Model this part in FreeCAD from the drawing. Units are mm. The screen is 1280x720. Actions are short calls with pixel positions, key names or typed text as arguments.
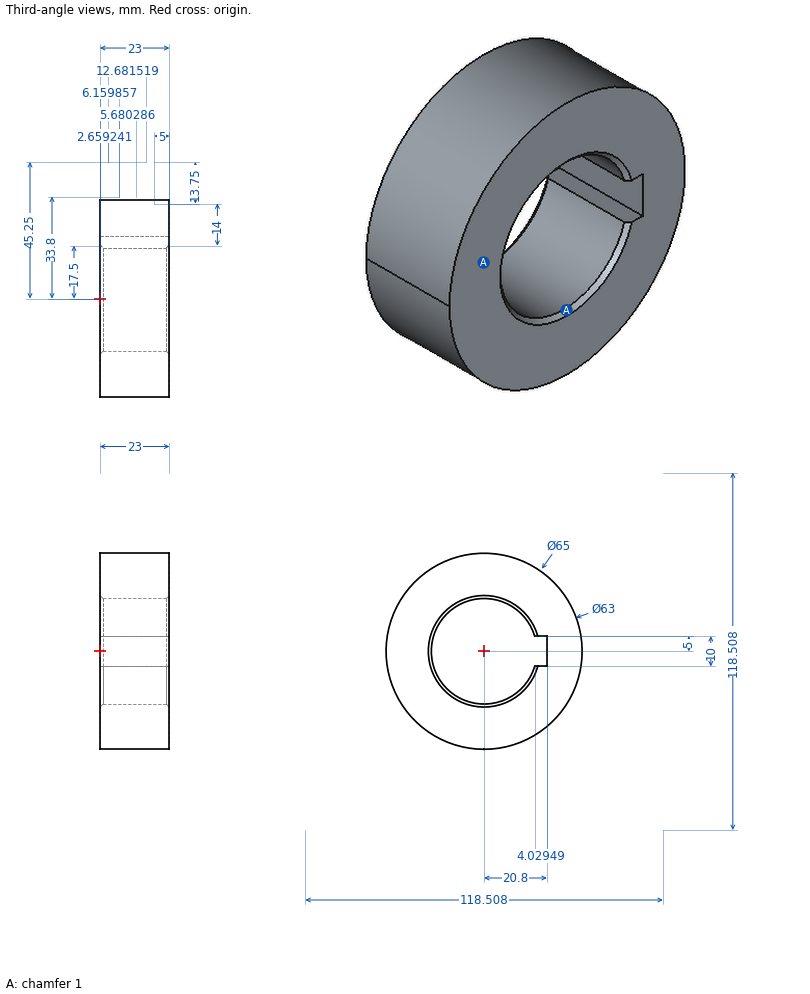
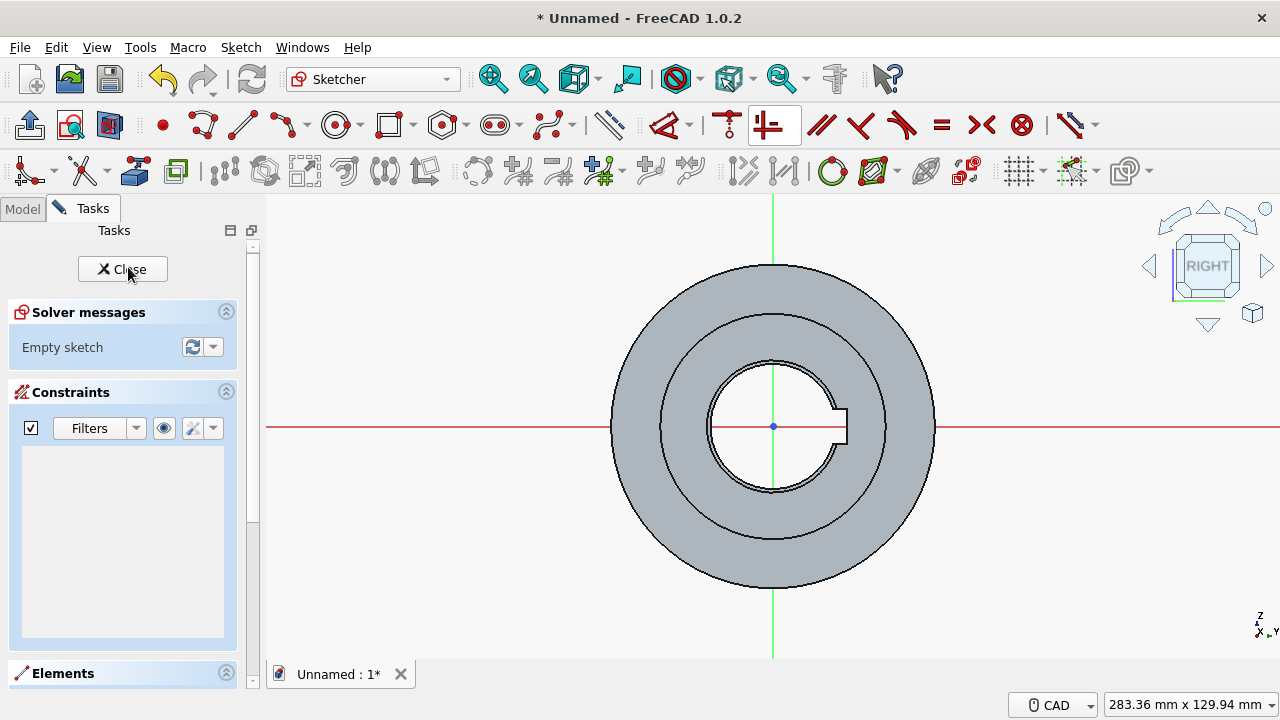
key(q)
key(s)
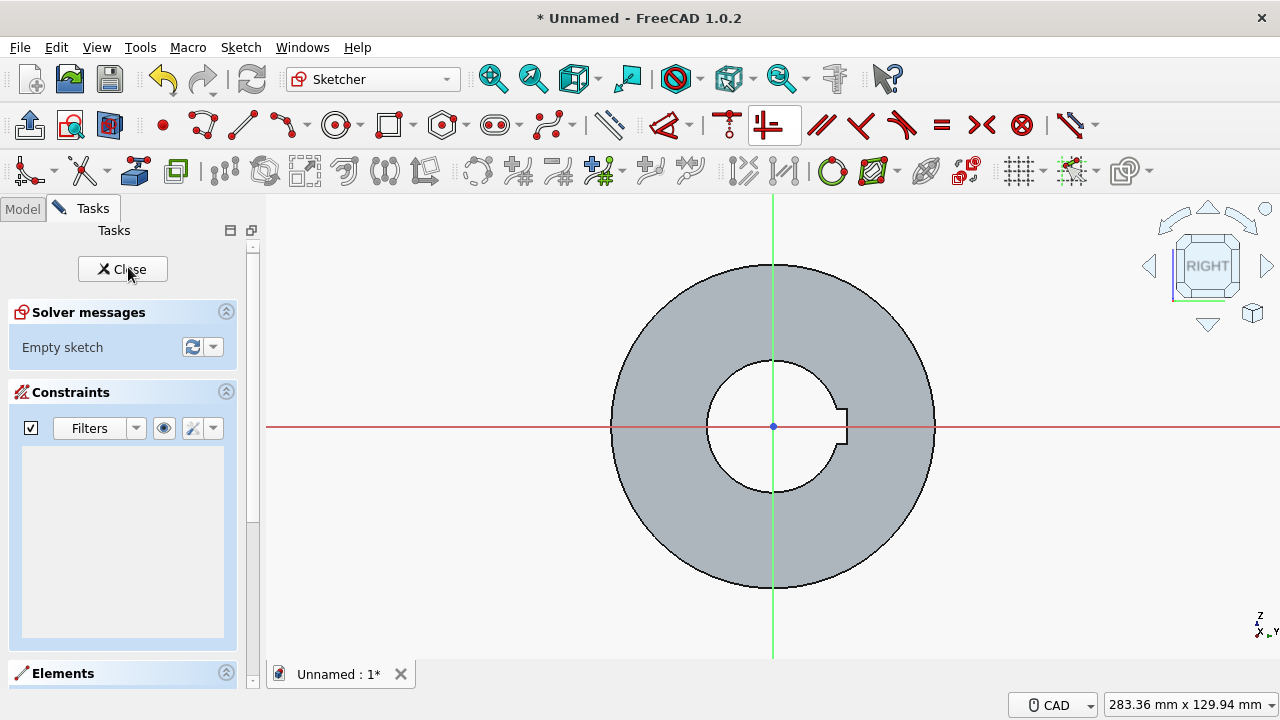
scroll(565, 426, down, 2)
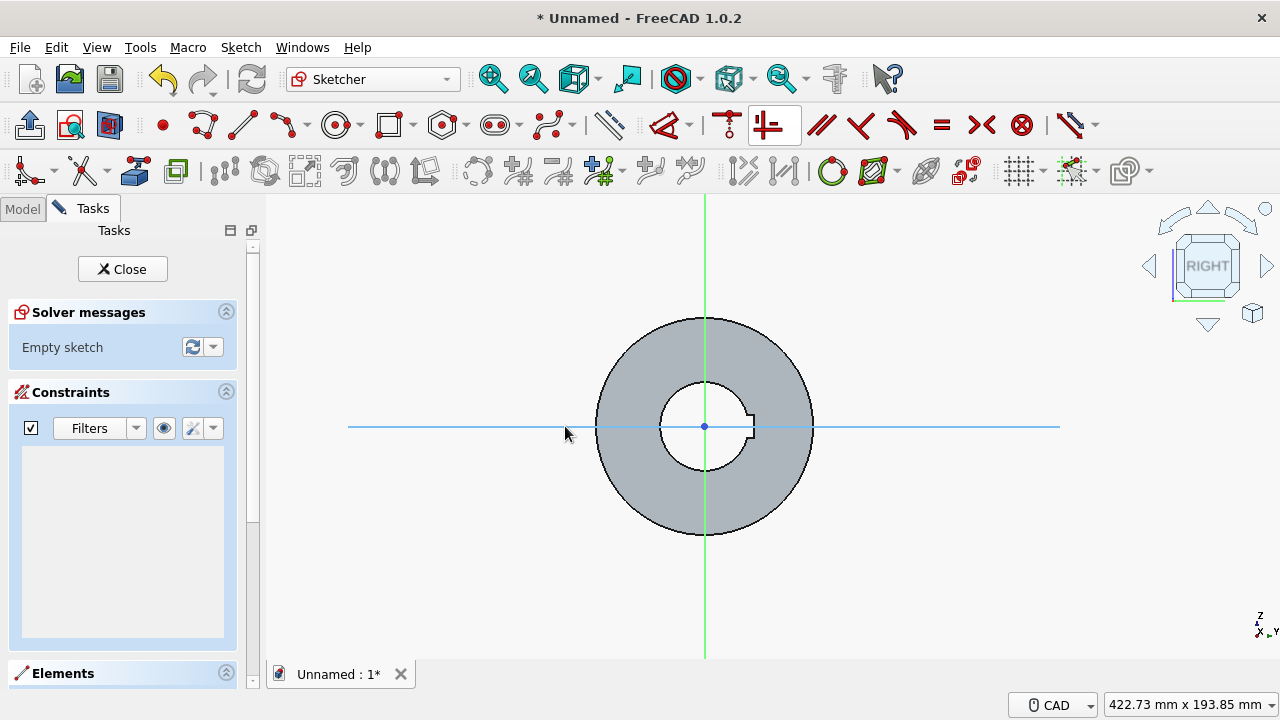
key(g)
key(v)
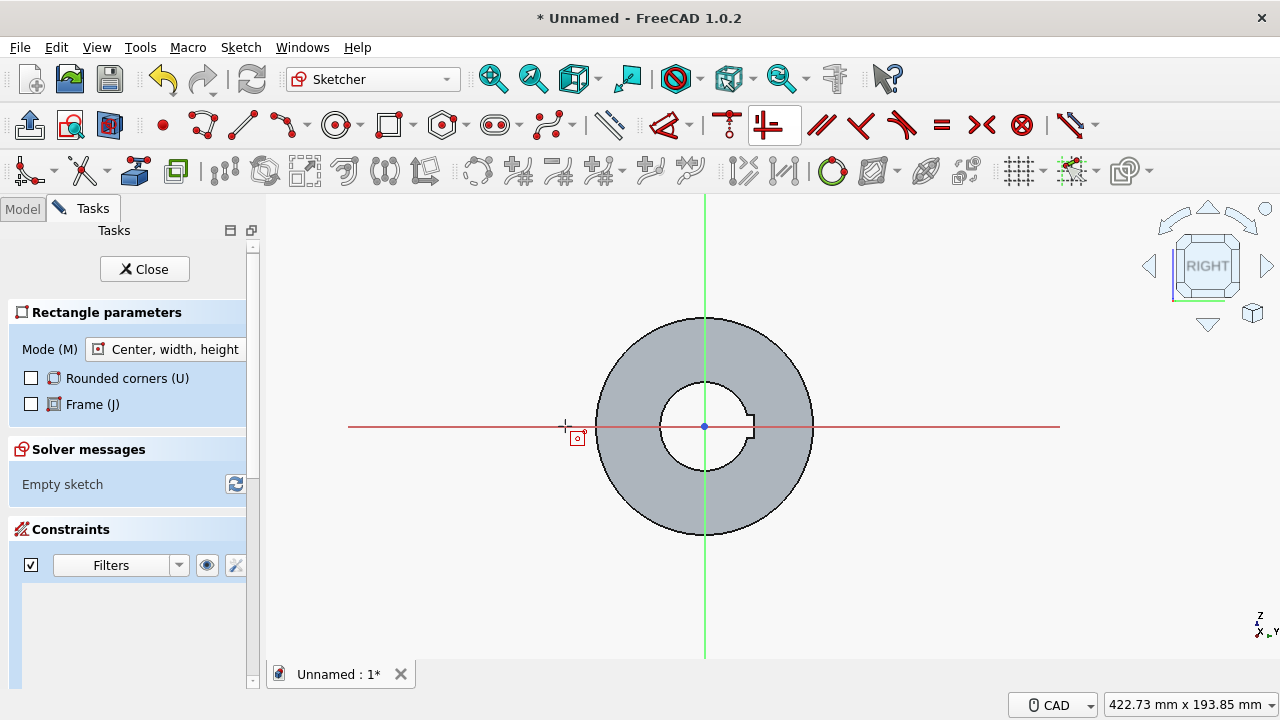
click(705, 427)
move(847, 284)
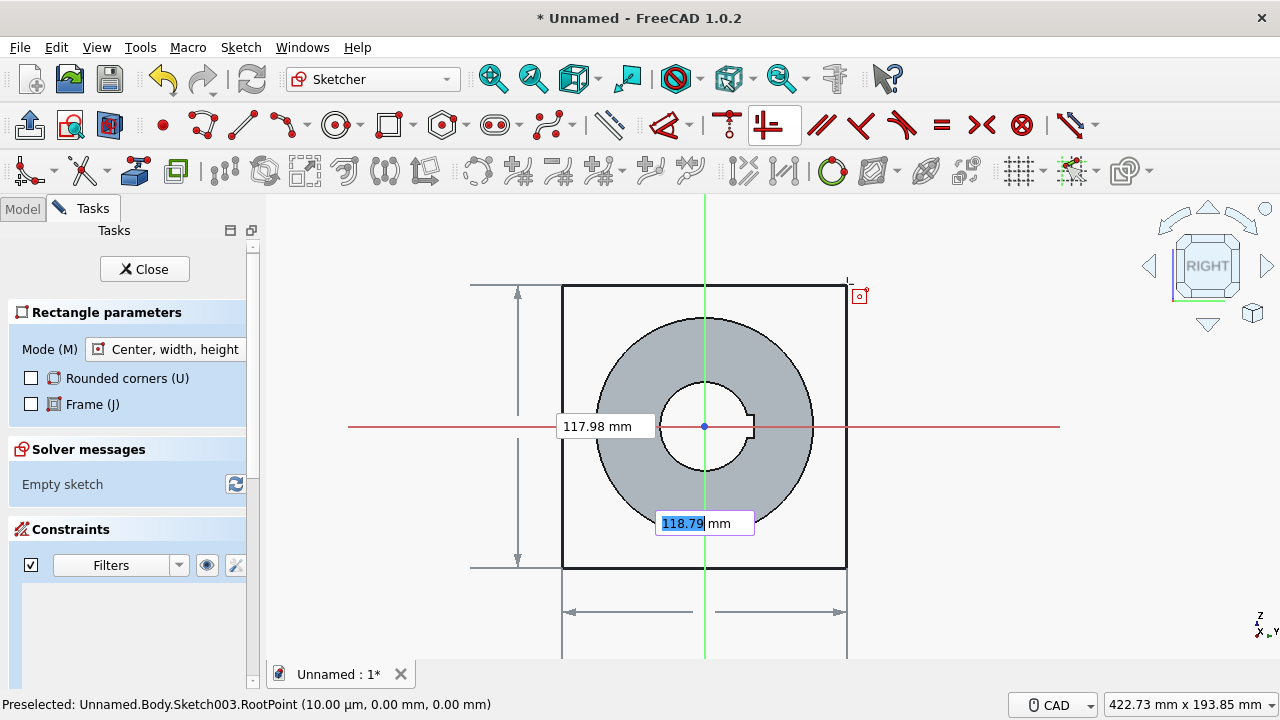
text(118.508)
key(Tab)
text(118.508)
key(Return)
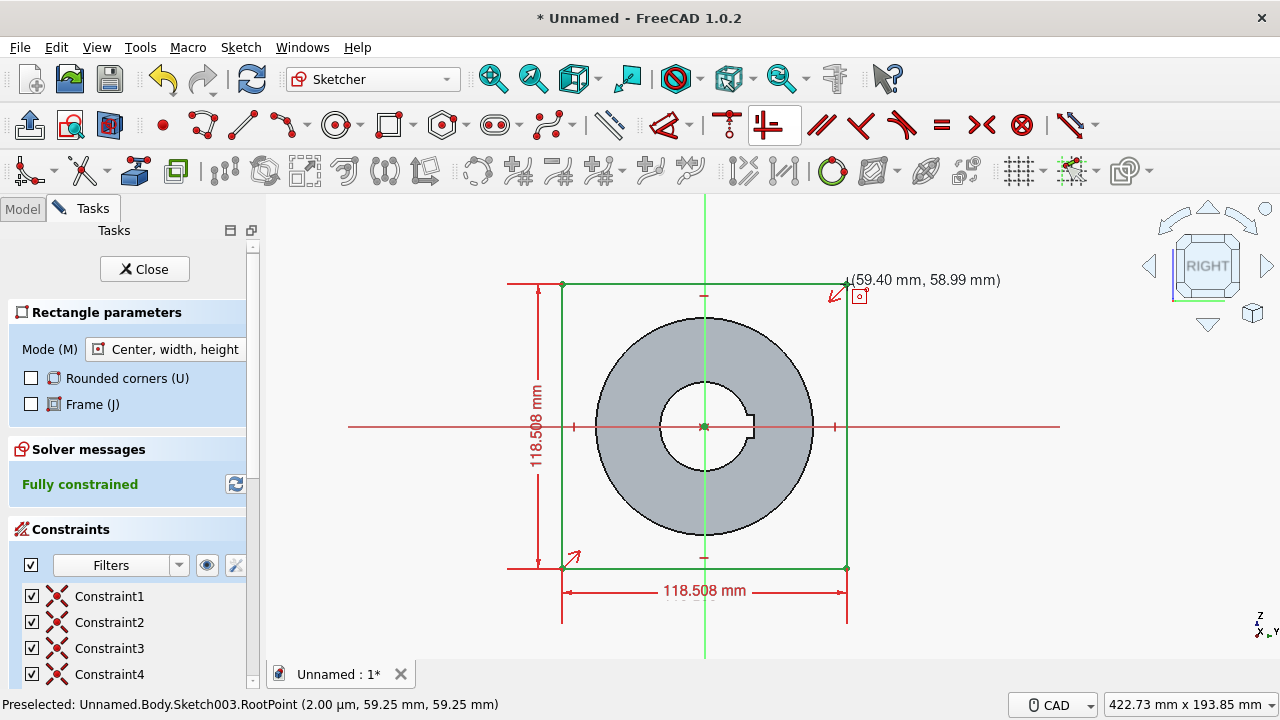
key(g)
key(c)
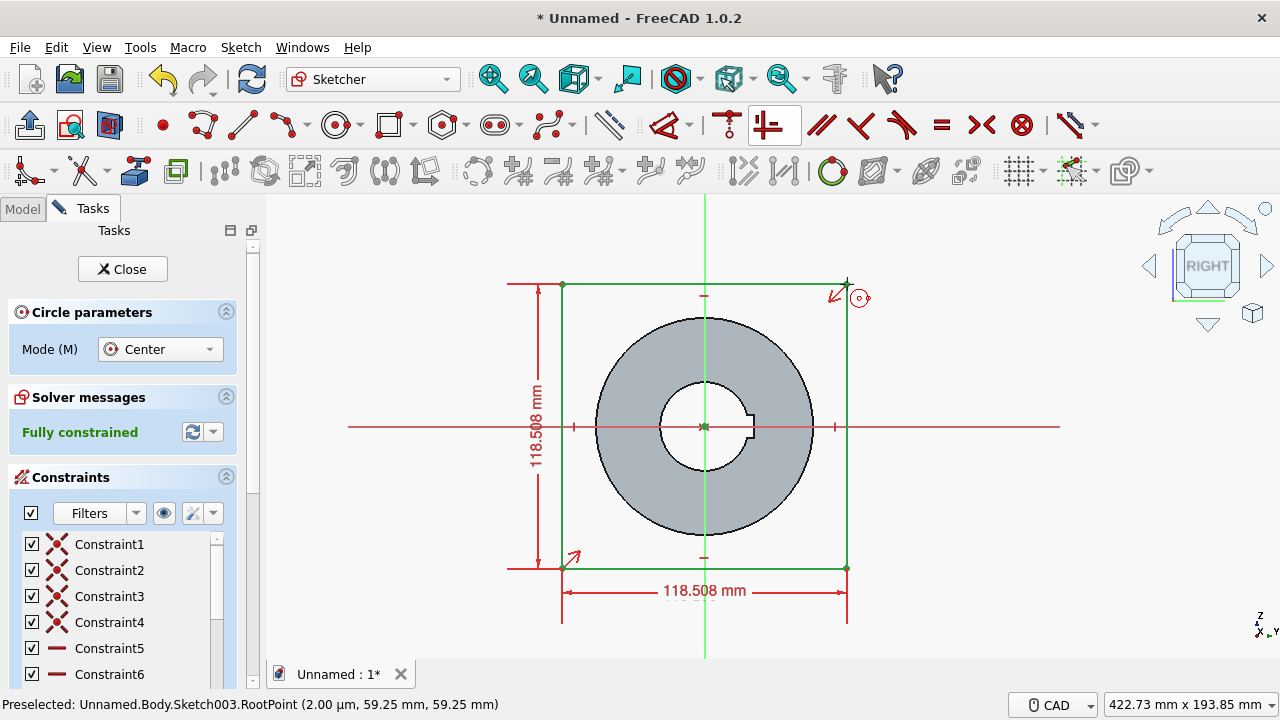
click(705, 427)
move(758, 373)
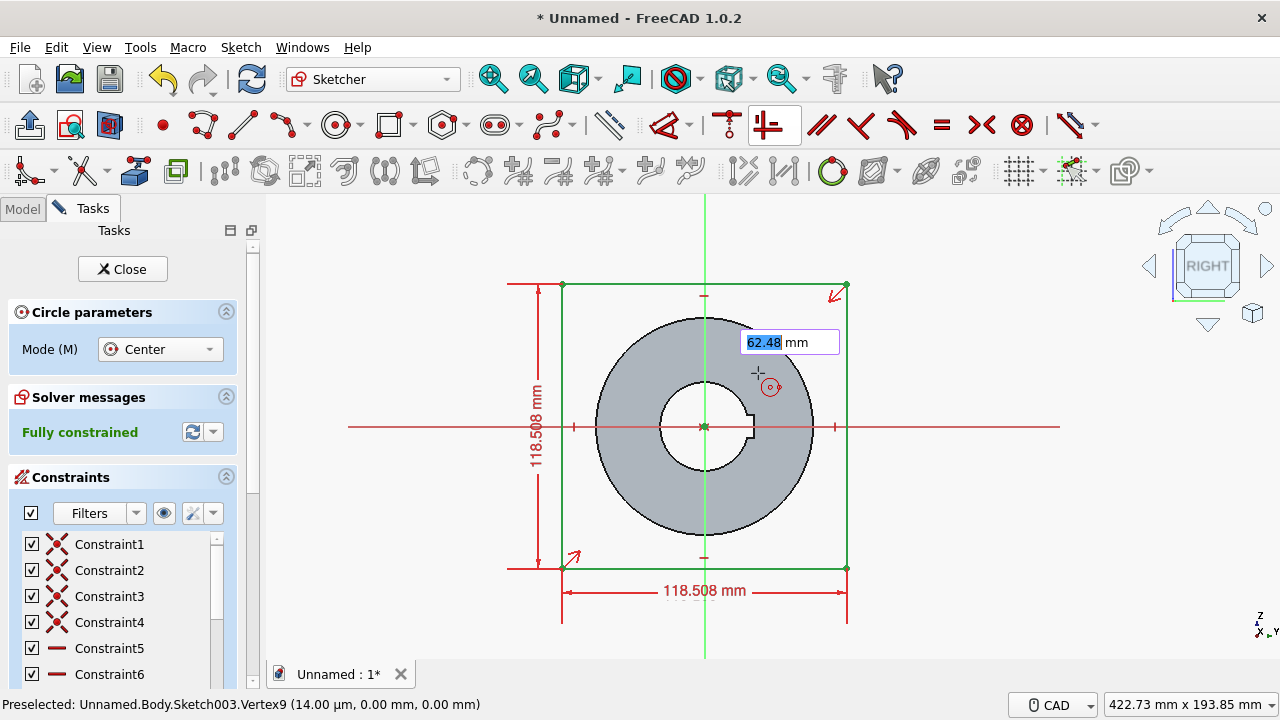
text(63)
key(Return)
key(Escape)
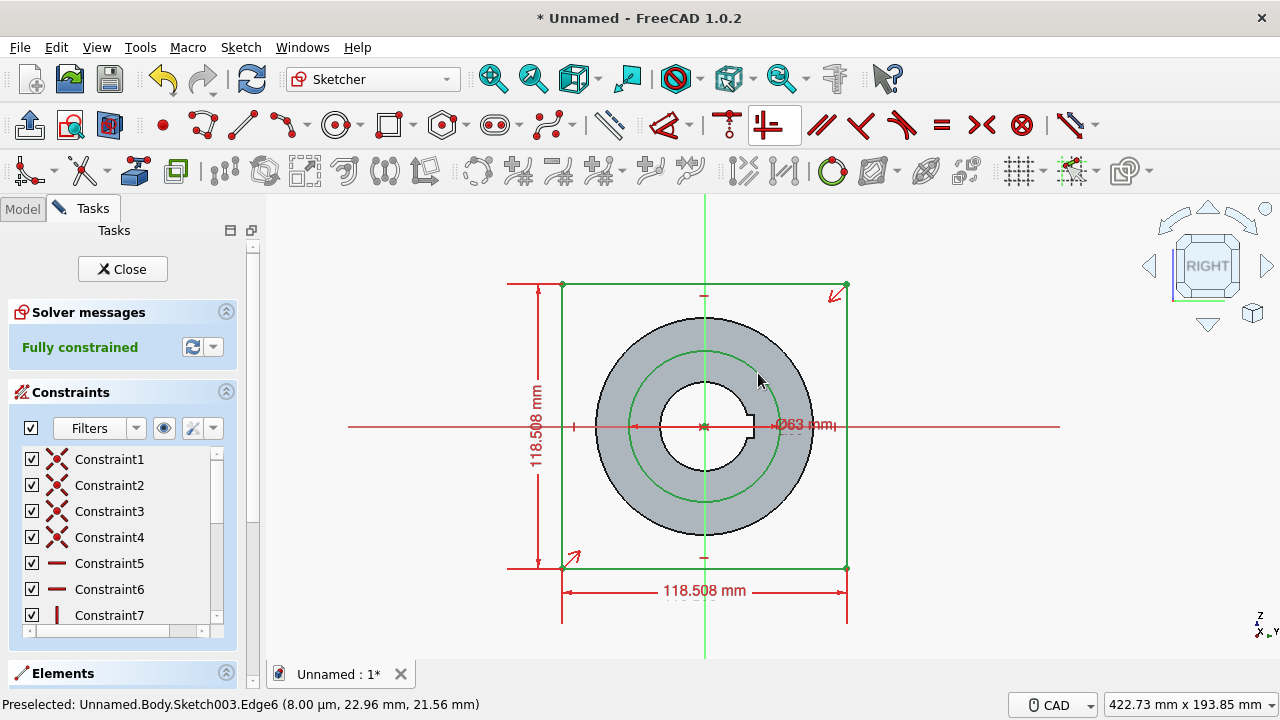
click(123, 269)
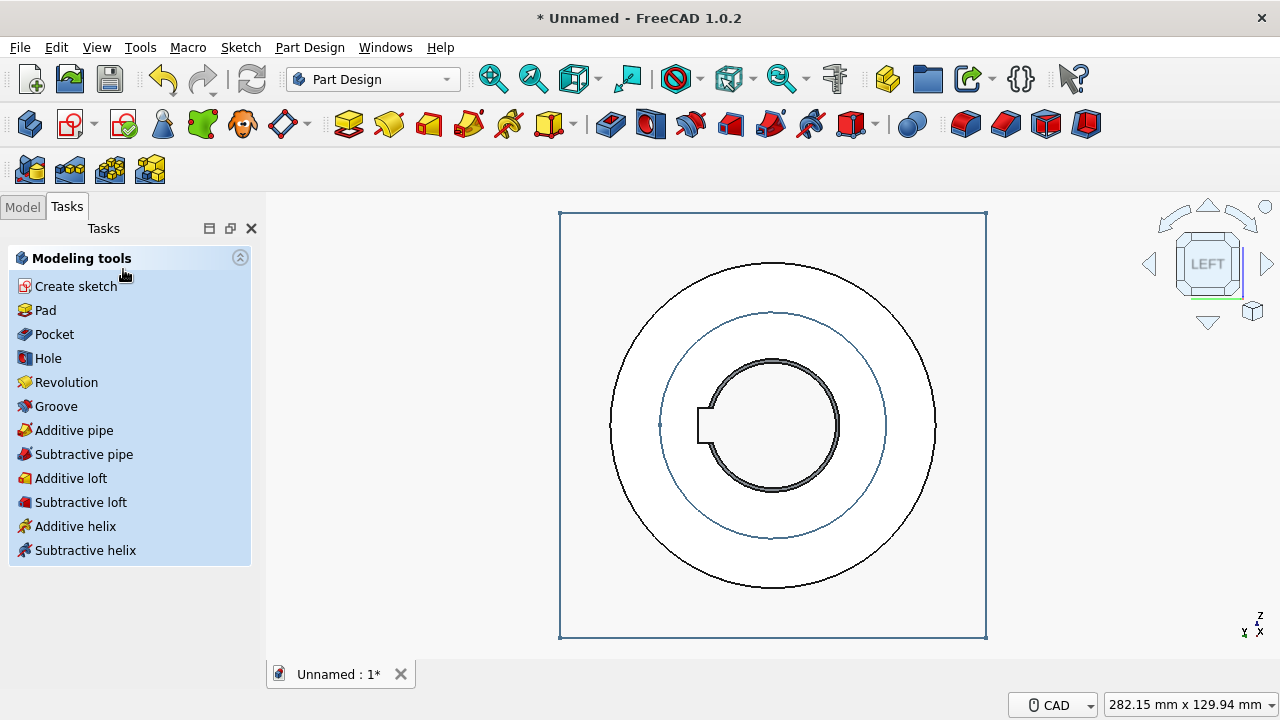
click(612, 124)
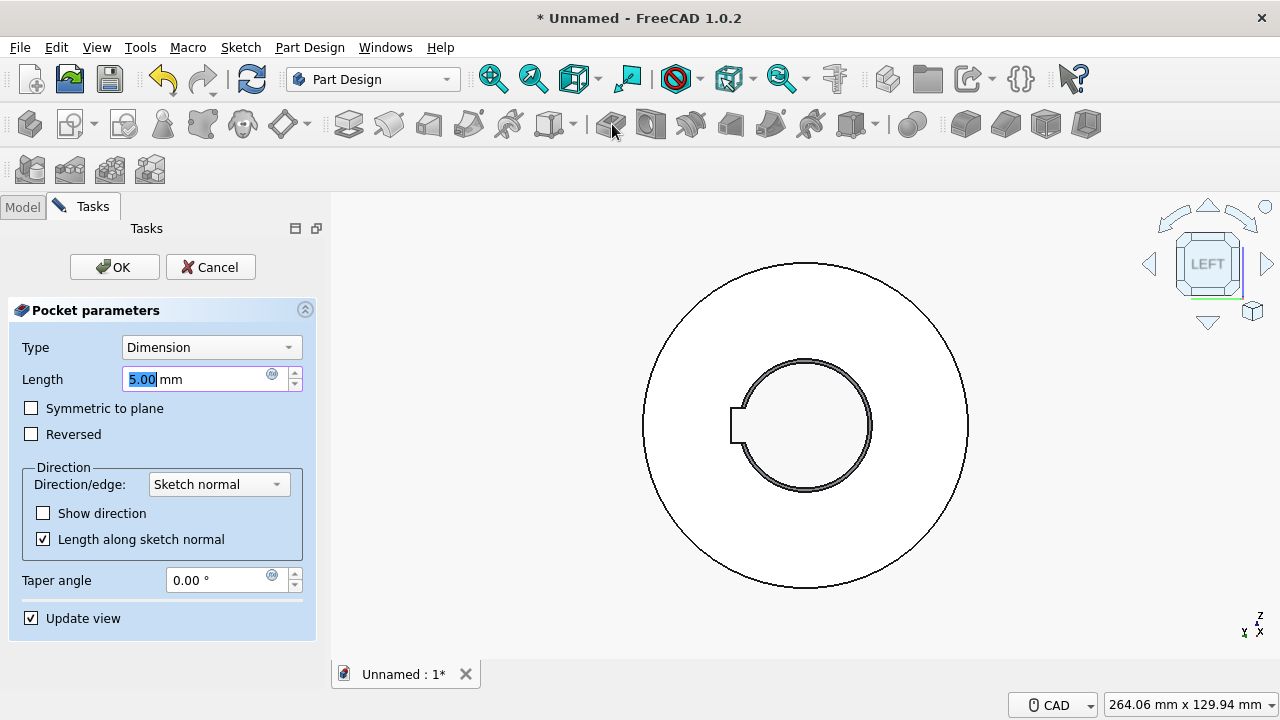
click(212, 348)